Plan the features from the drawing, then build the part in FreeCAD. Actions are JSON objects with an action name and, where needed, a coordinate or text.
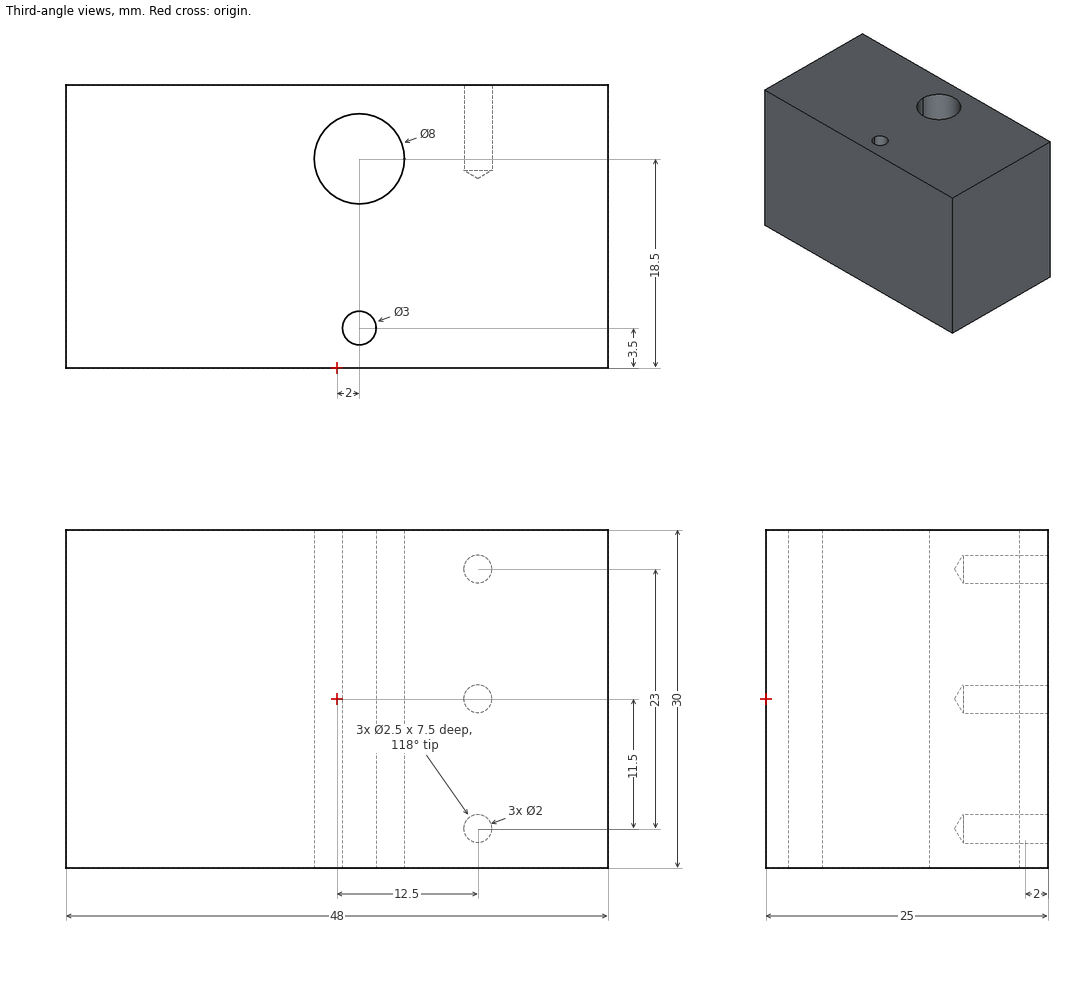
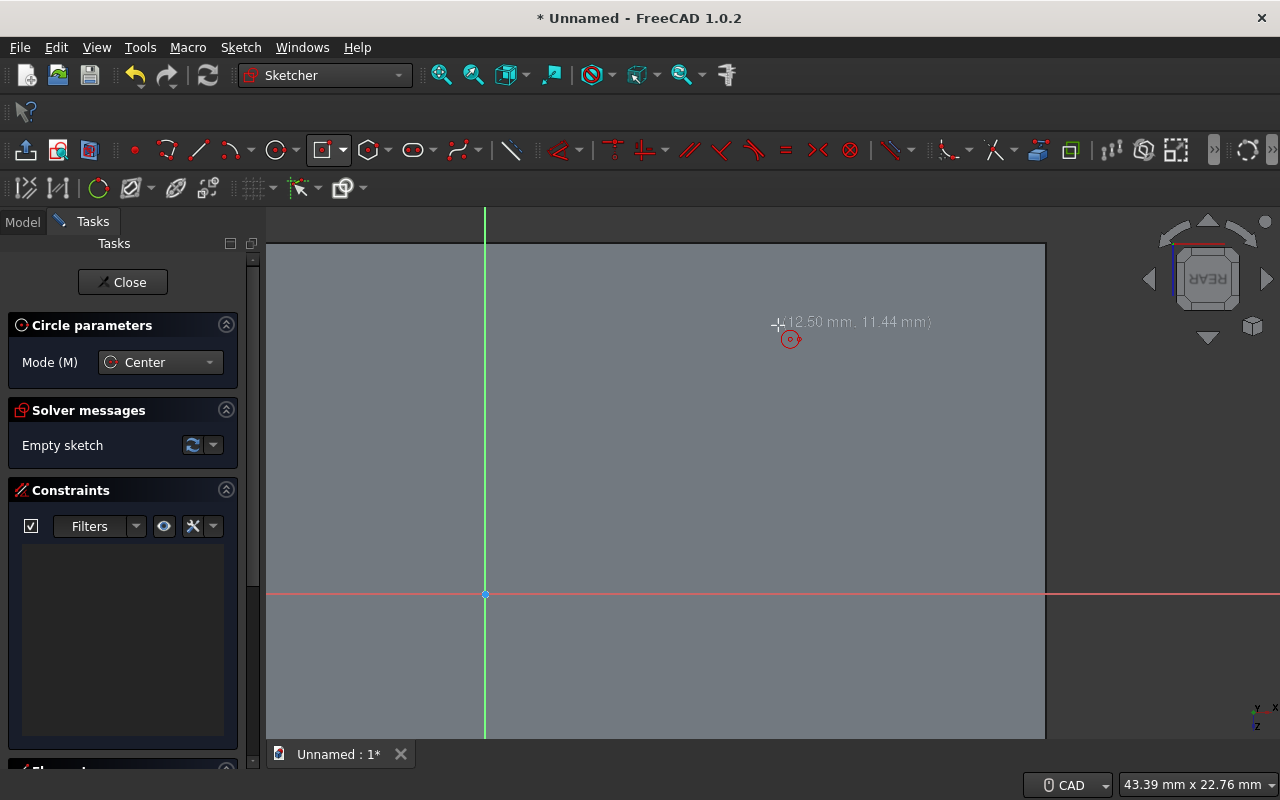
{"action": "left_click", "coordinate": [778, 325]}
{"action": "left_click", "coordinate": [794, 309]}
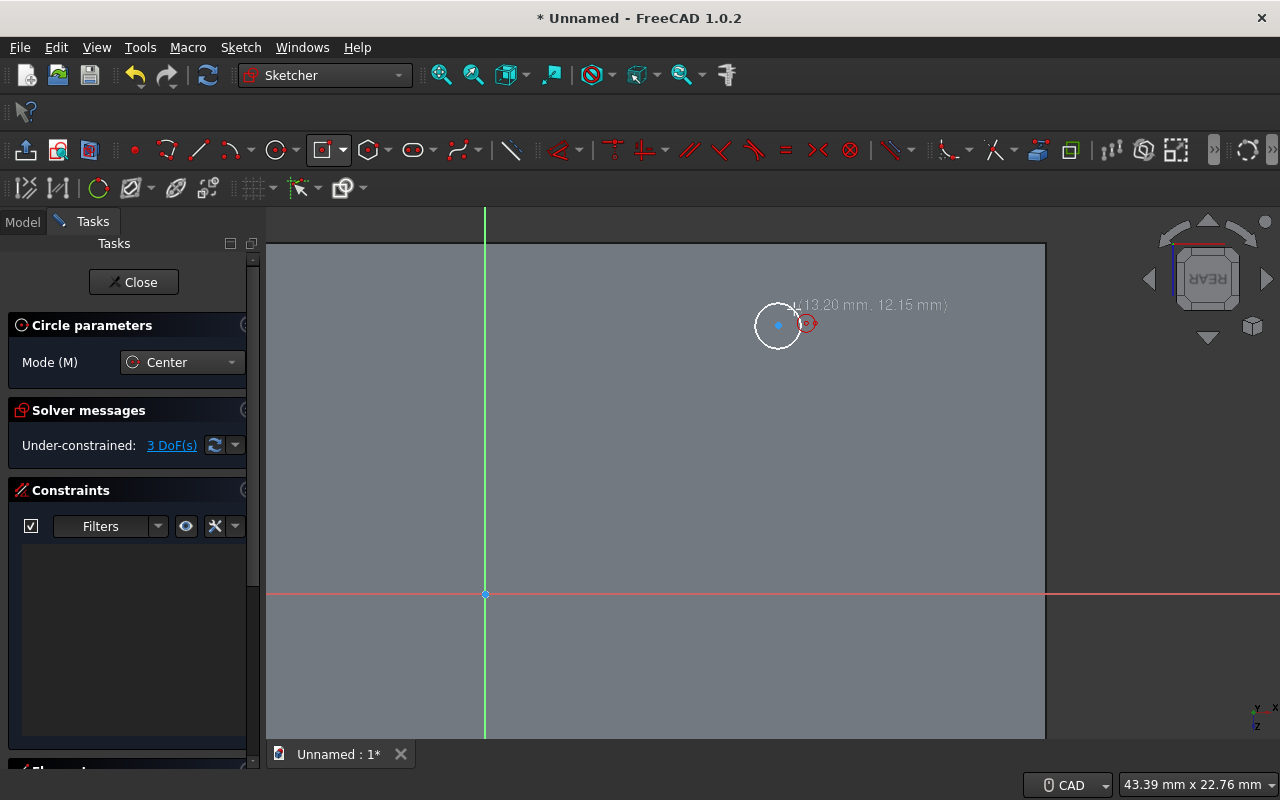
{"action": "left_click", "coordinate": [778, 594]}
{"action": "left_click", "coordinate": [794, 578]}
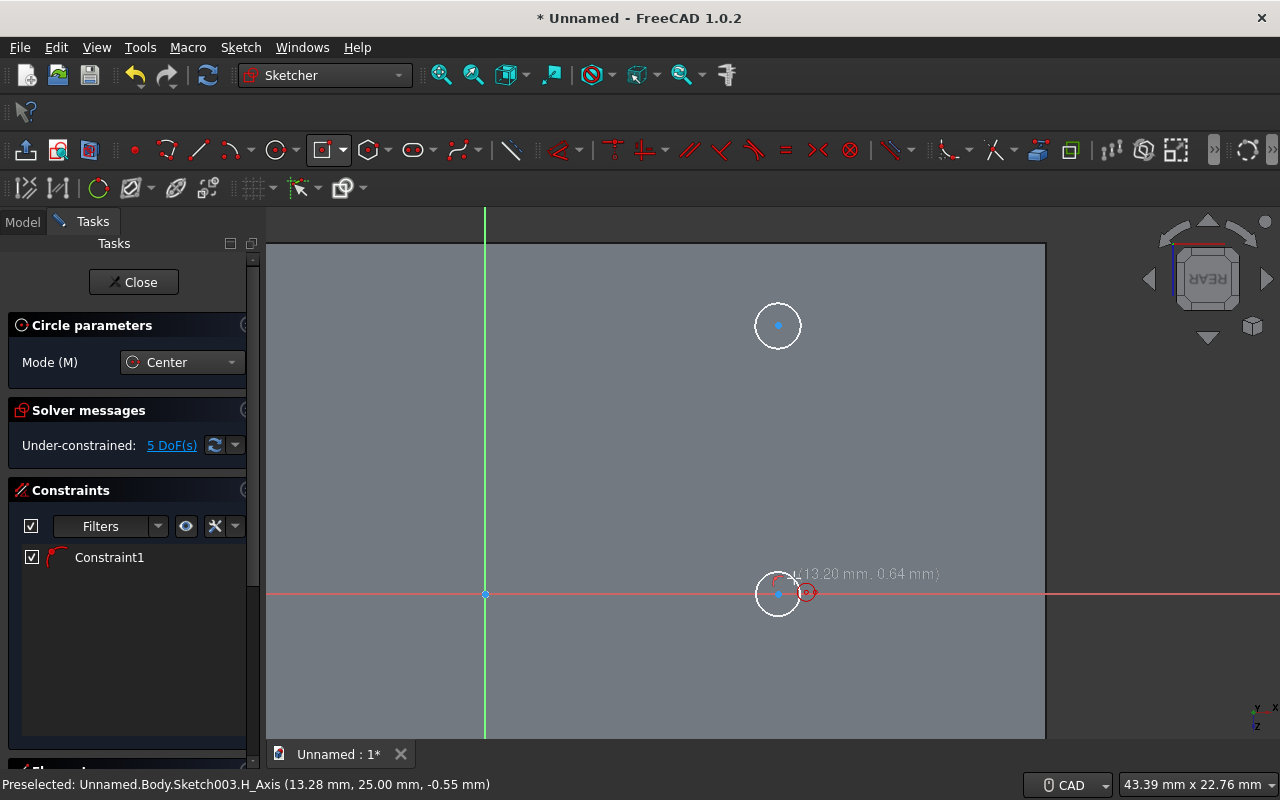
{"action": "scroll", "coordinate": [779, 326], "scroll_direction": "down", "scroll_amount": 3}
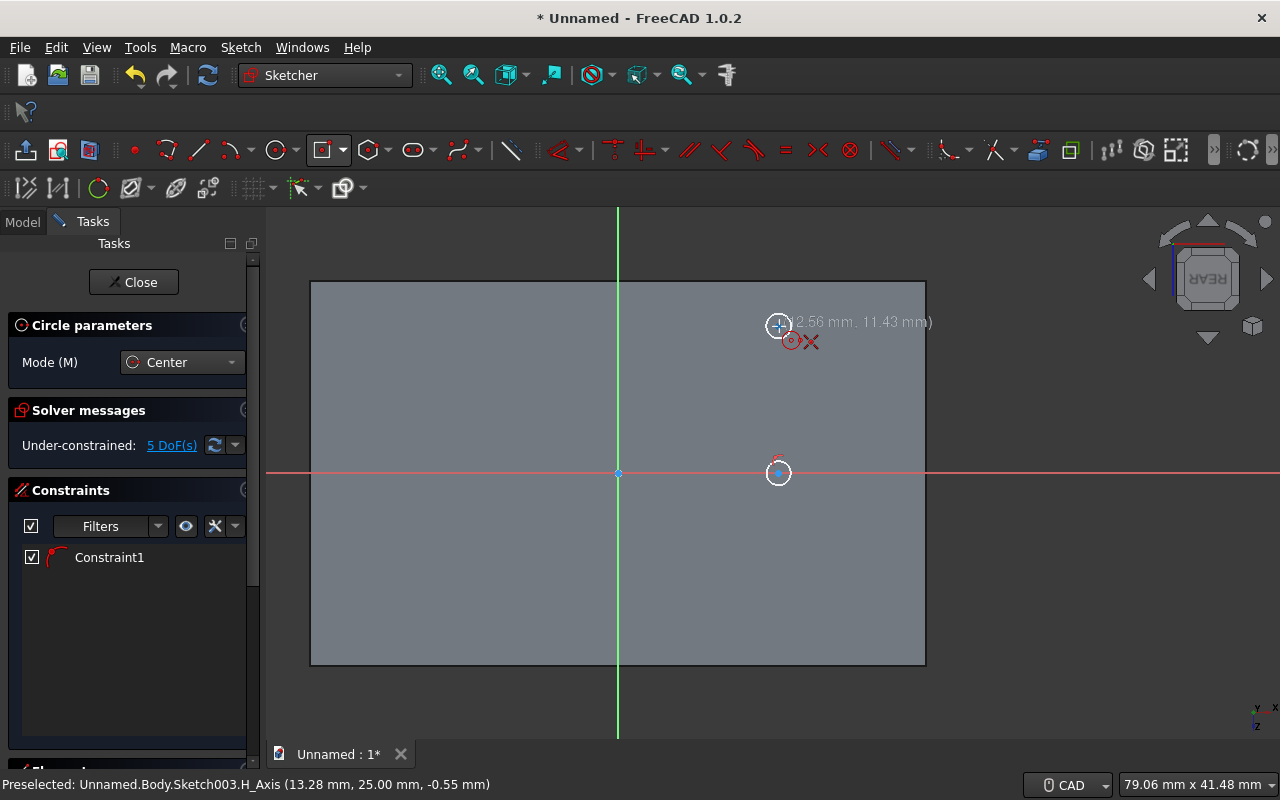
{"action": "scroll", "coordinate": [778, 621], "scroll_direction": "up", "scroll_amount": 3}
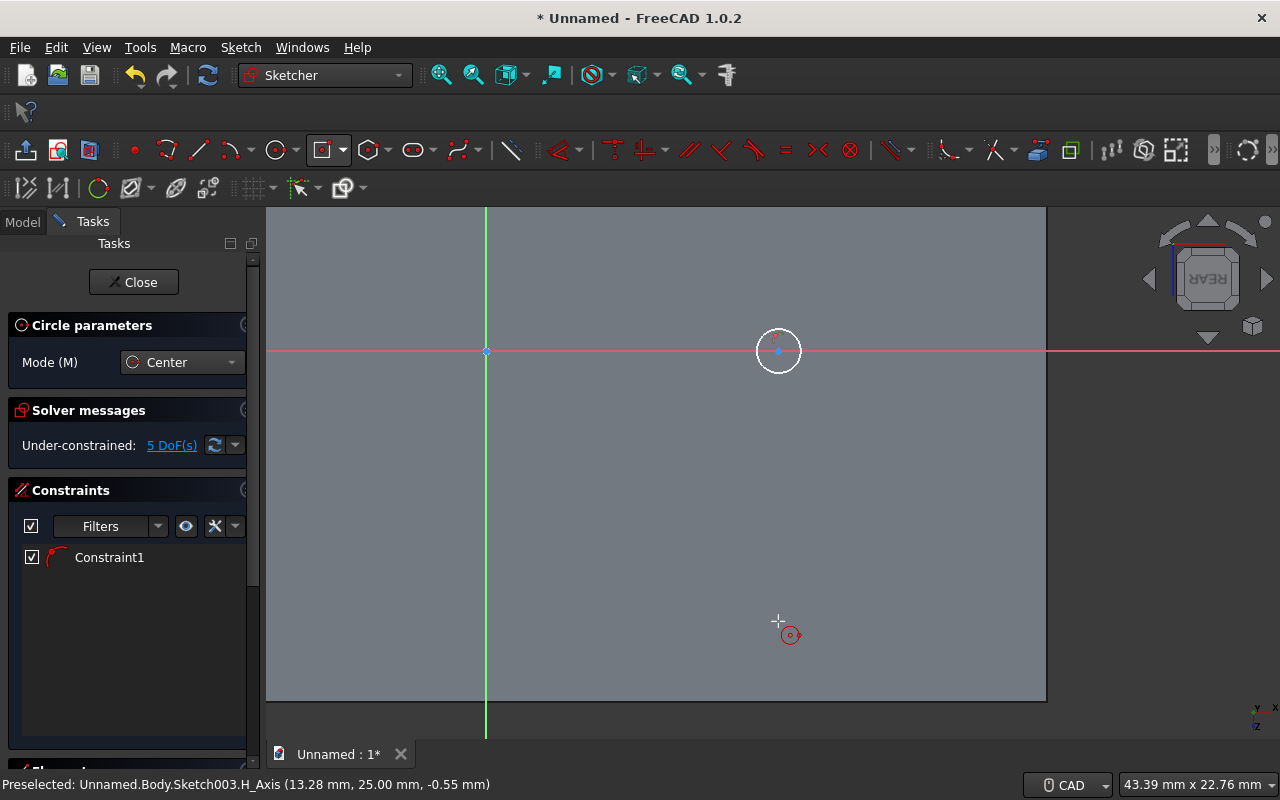
{"action": "left_click", "coordinate": [778, 620]}
{"action": "left_click", "coordinate": [795, 603]}
{"action": "key", "text": "Escape"}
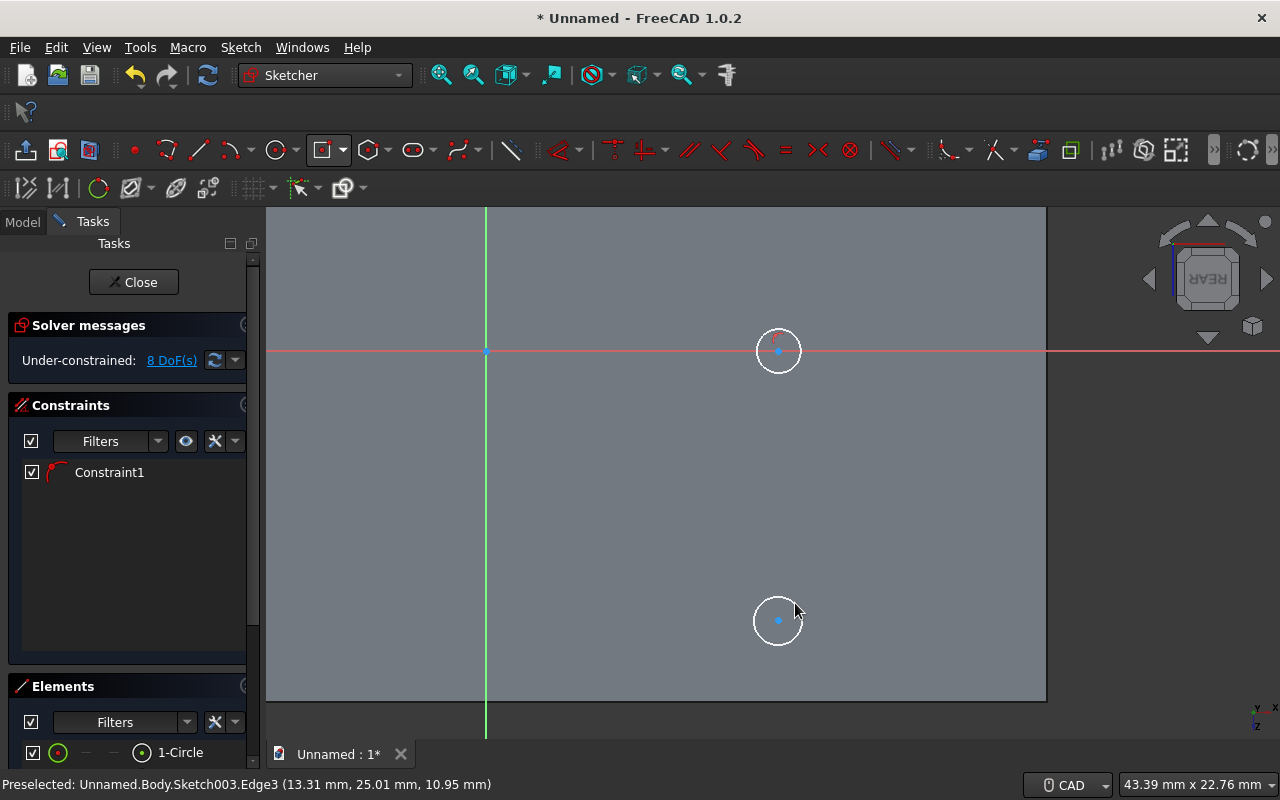
{"action": "scroll", "coordinate": [778, 621], "scroll_direction": "down", "scroll_amount": 3}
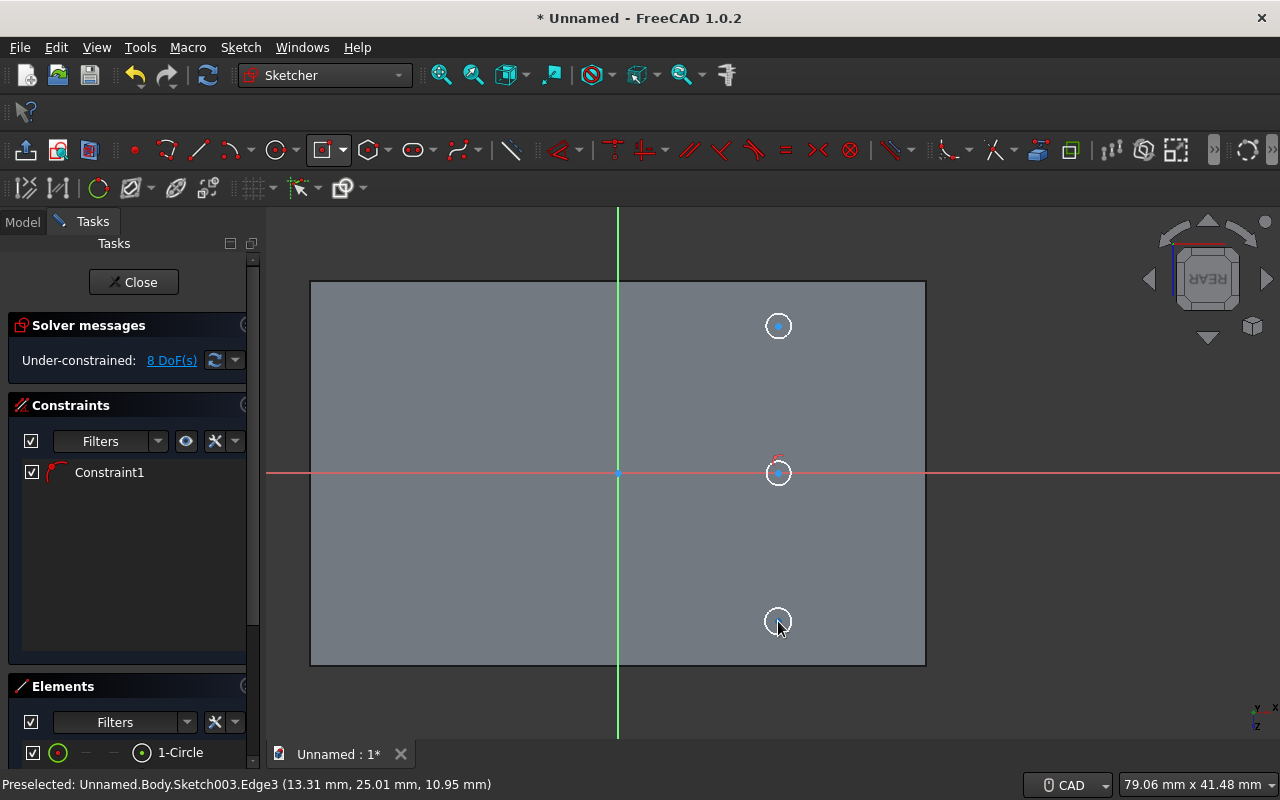
{"action": "left_click", "coordinate": [787, 317]}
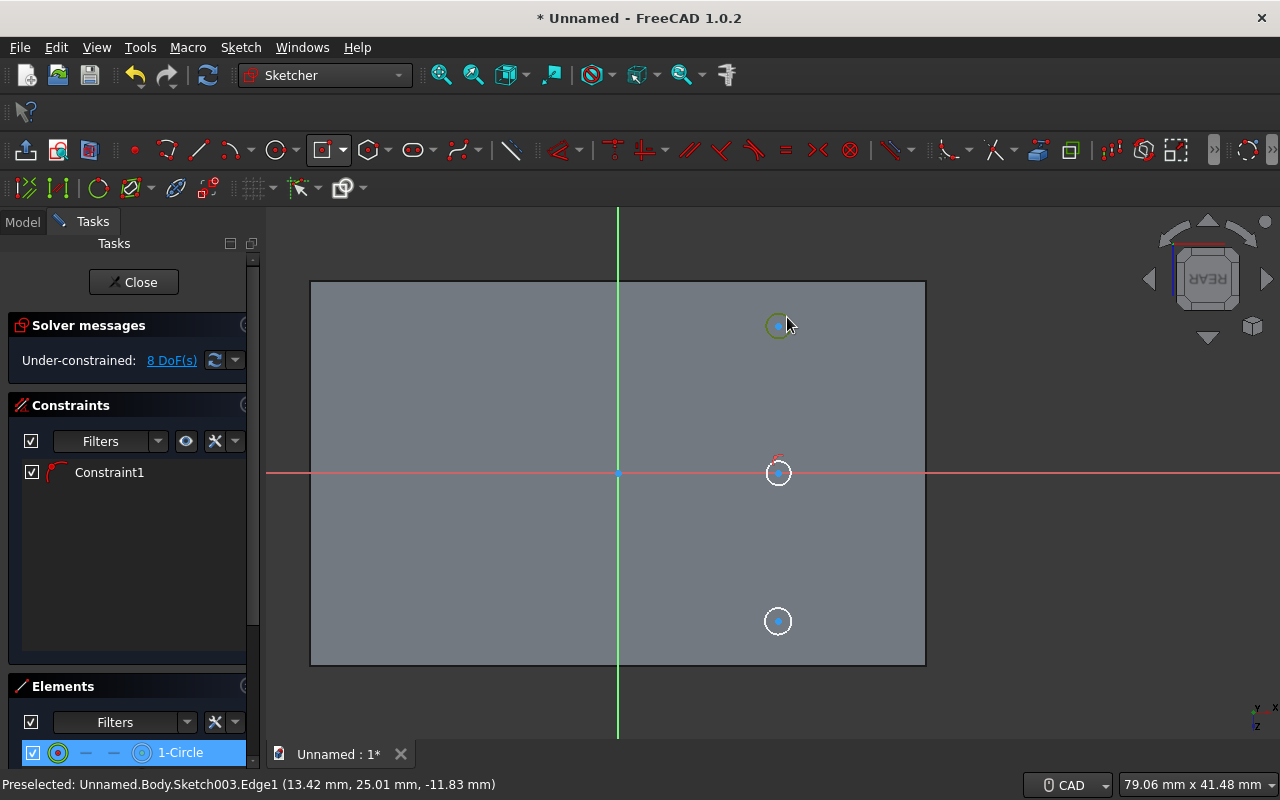
{"action": "left_click", "coordinate": [767, 473]}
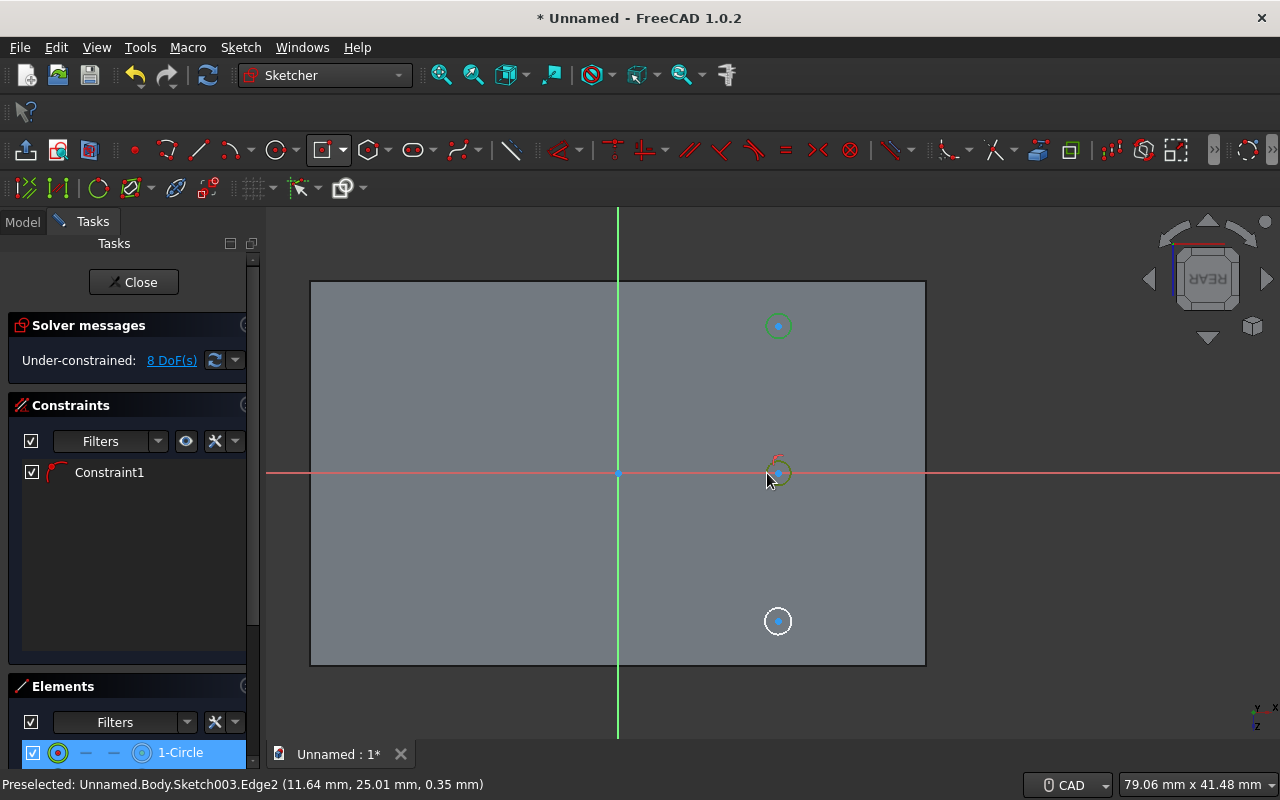
{"action": "left_click", "coordinate": [788, 612]}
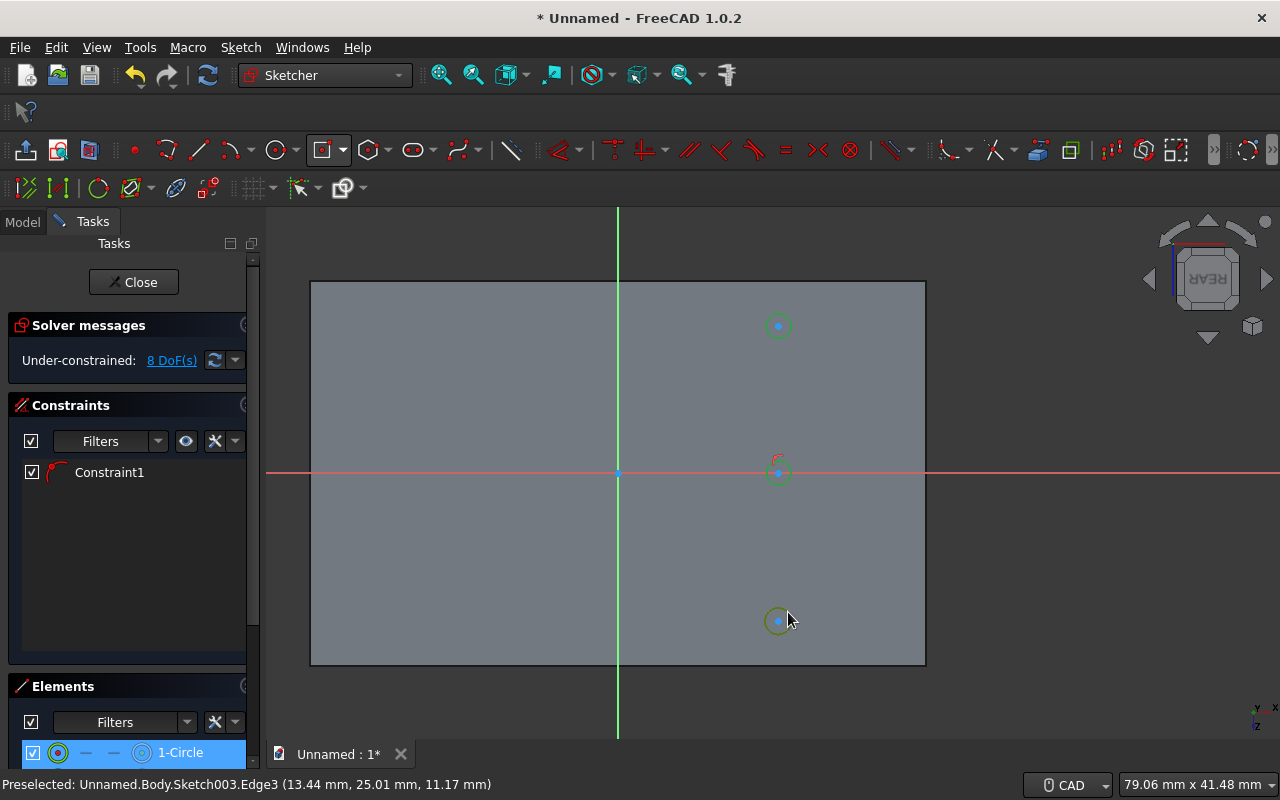
{"action": "key", "text": "e"}